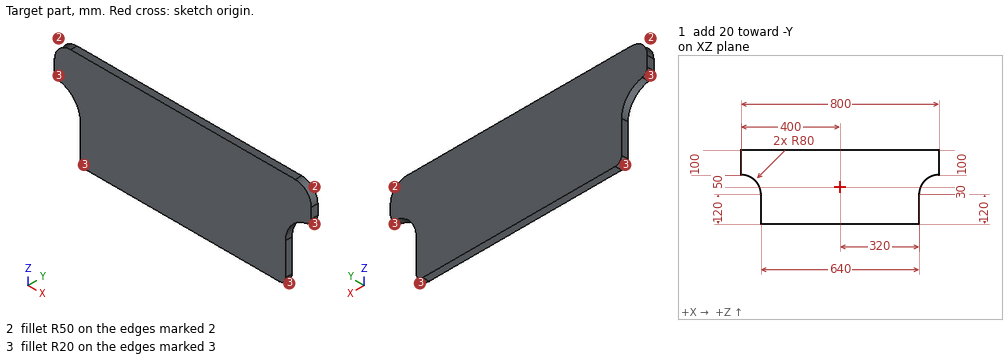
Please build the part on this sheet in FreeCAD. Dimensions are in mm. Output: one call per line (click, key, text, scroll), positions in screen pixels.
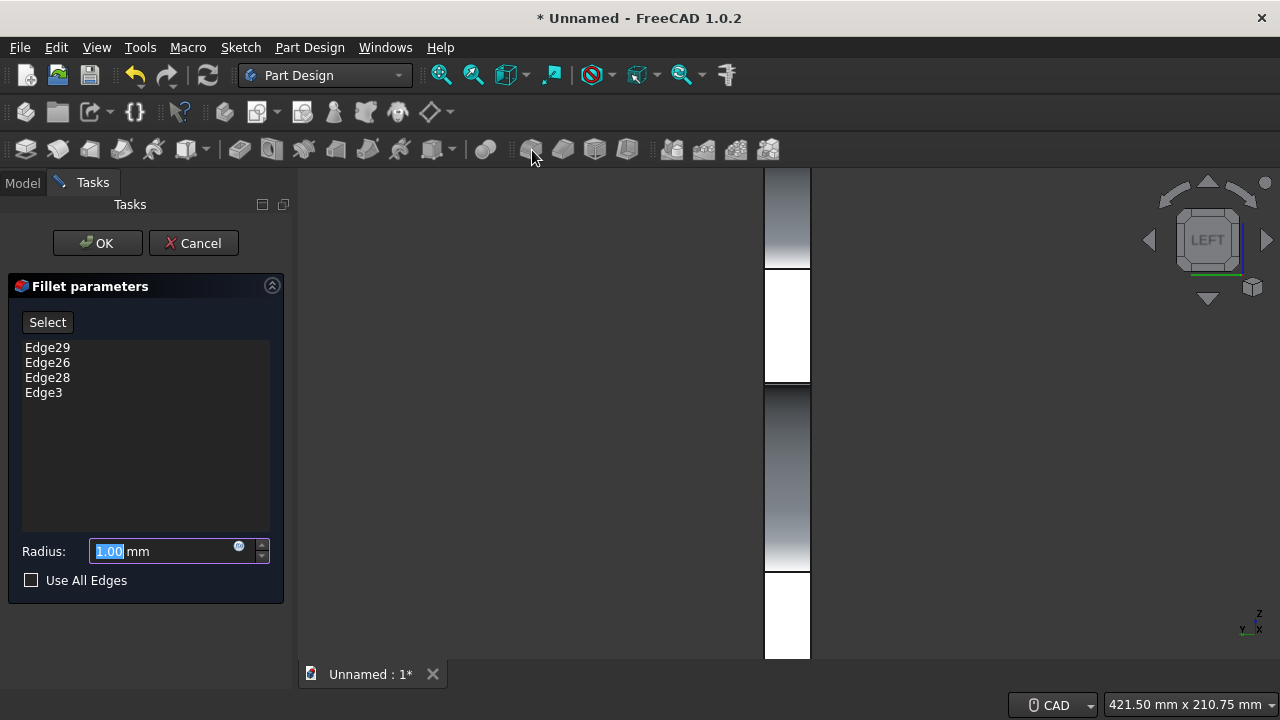
text(20)
key(Tab)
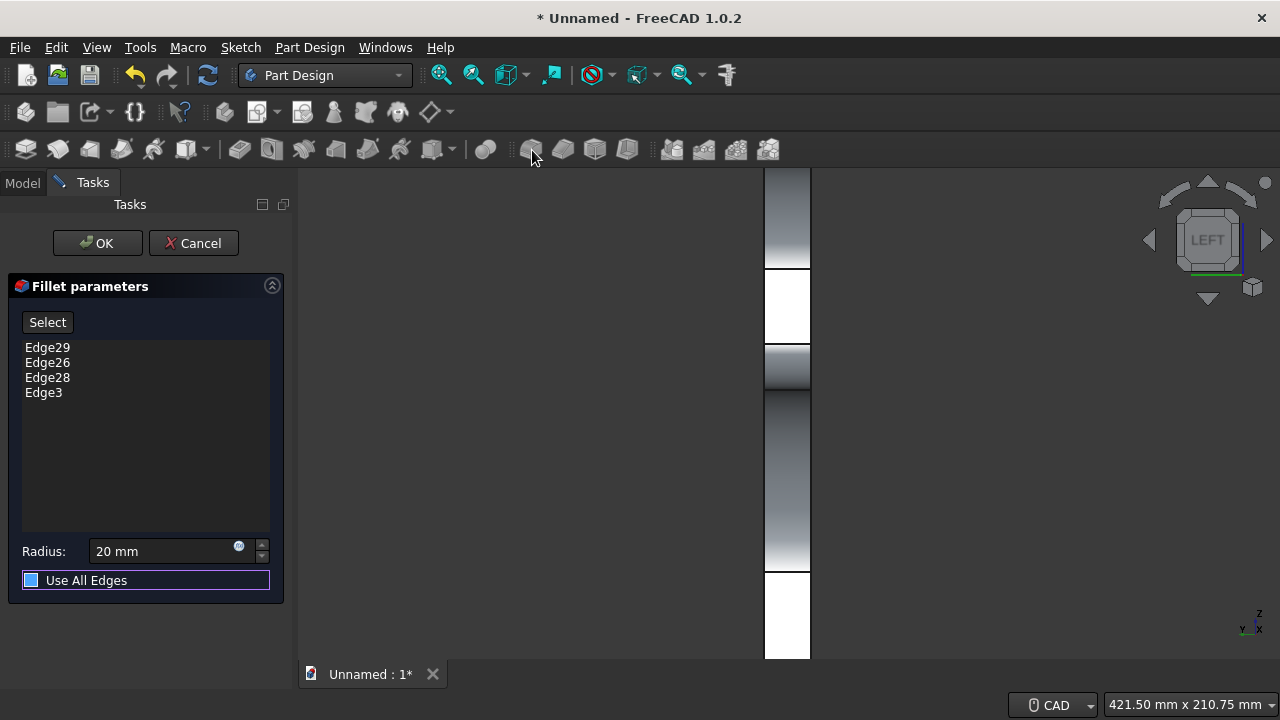
click(98, 243)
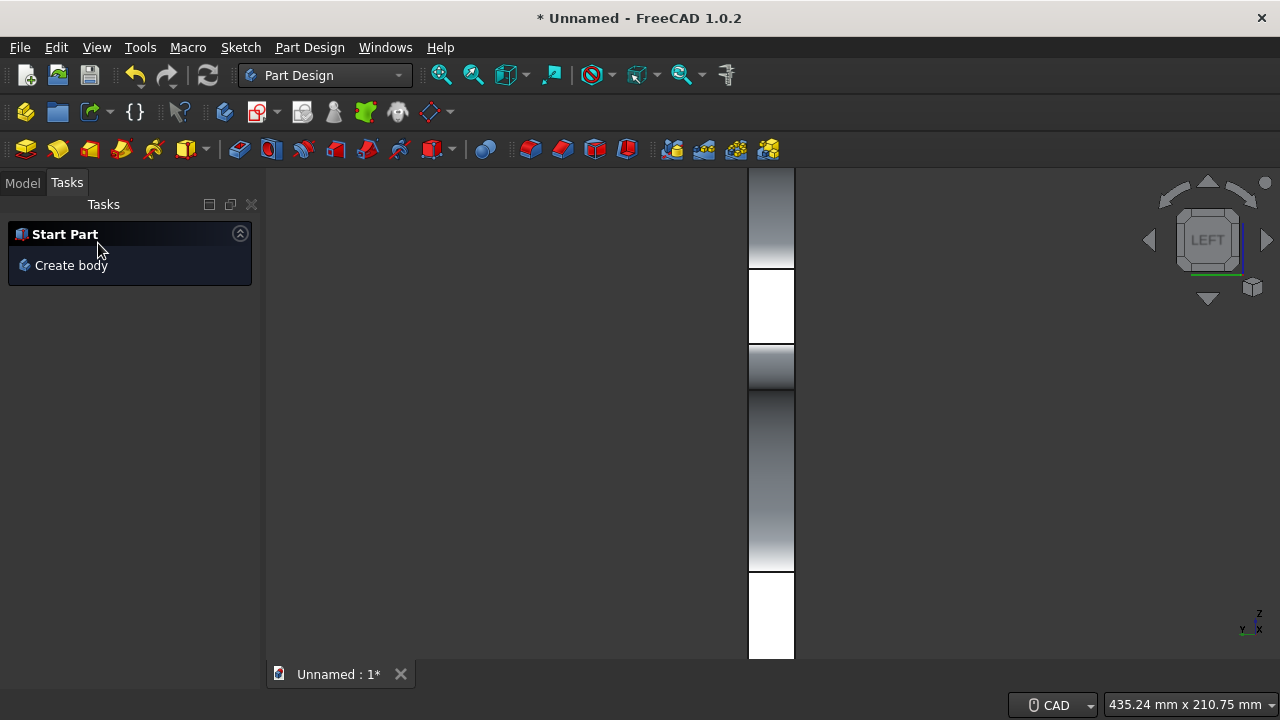
key(0)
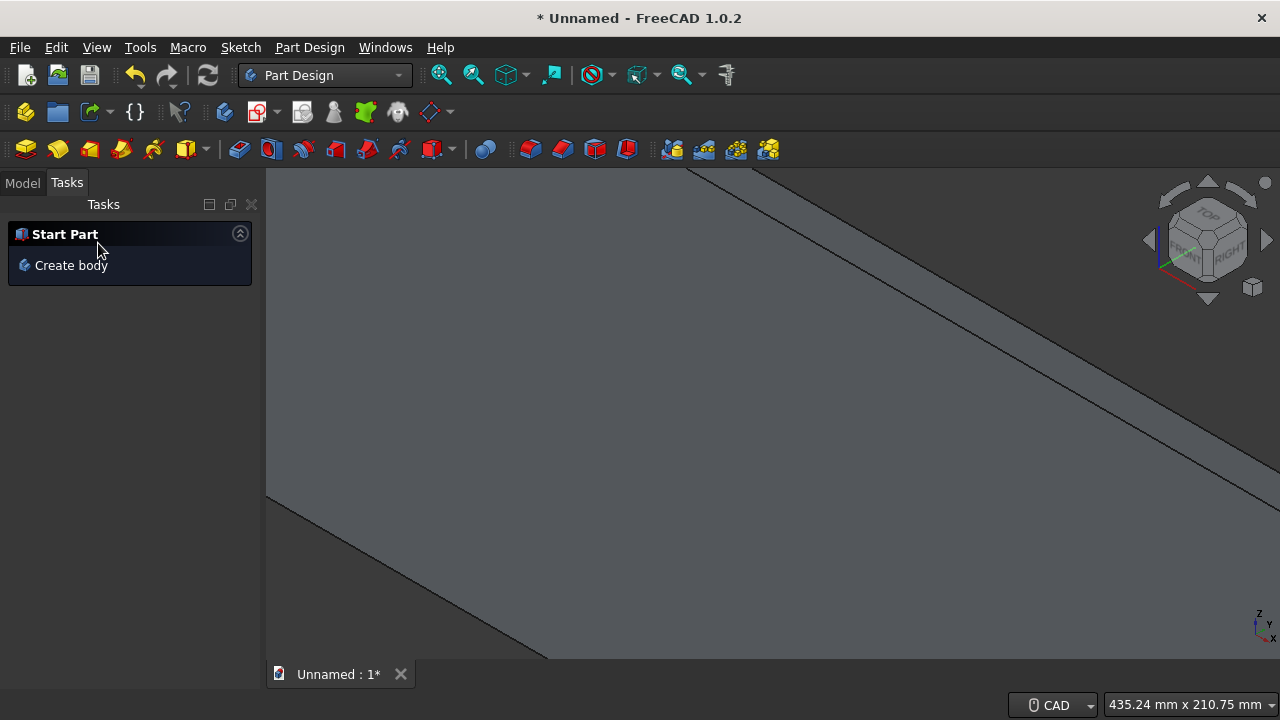
key(v)
key(f)